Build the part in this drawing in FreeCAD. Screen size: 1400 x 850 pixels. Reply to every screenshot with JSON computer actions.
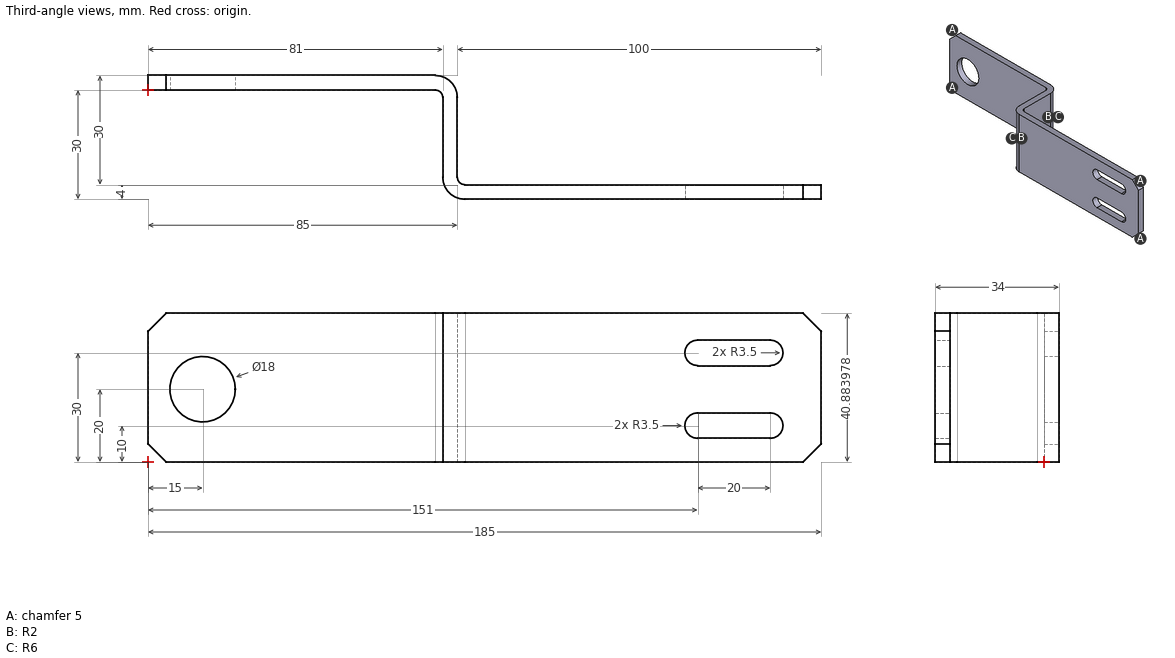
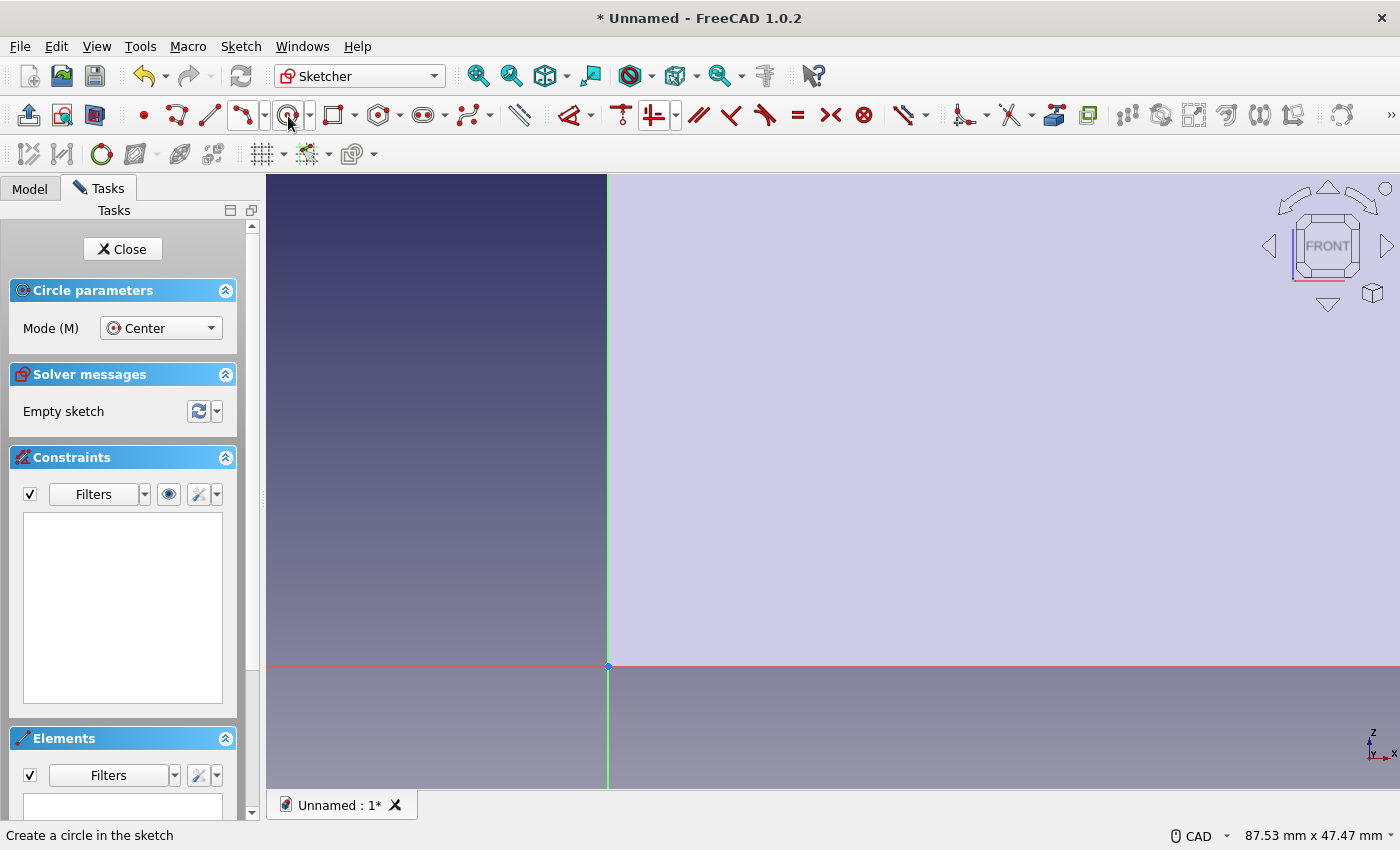
{"action": "left_click", "coordinate": [803, 408]}
{"action": "left_click", "coordinate": [885, 325]}
{"action": "key", "text": "Escape"}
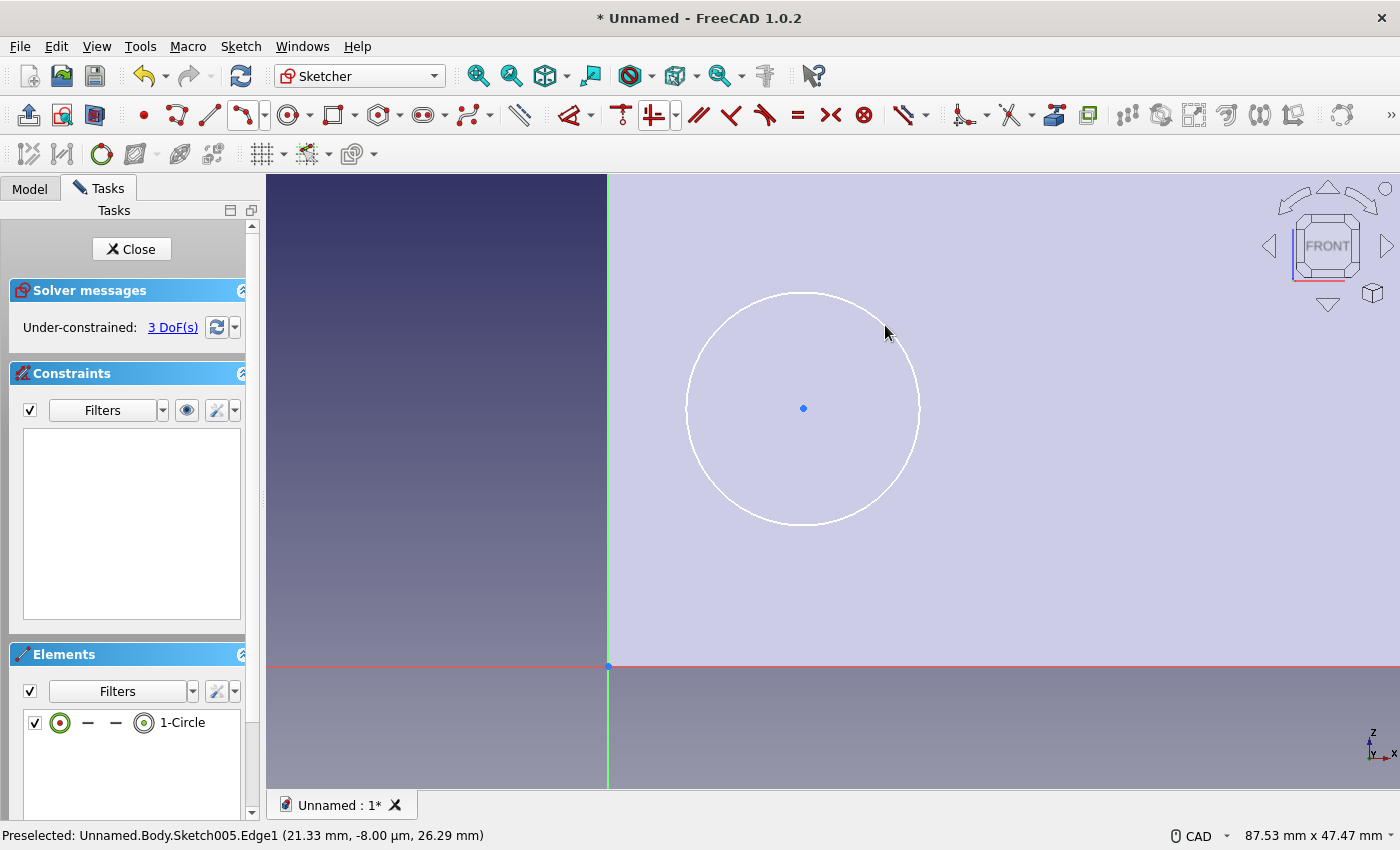
{"action": "key", "text": "d"}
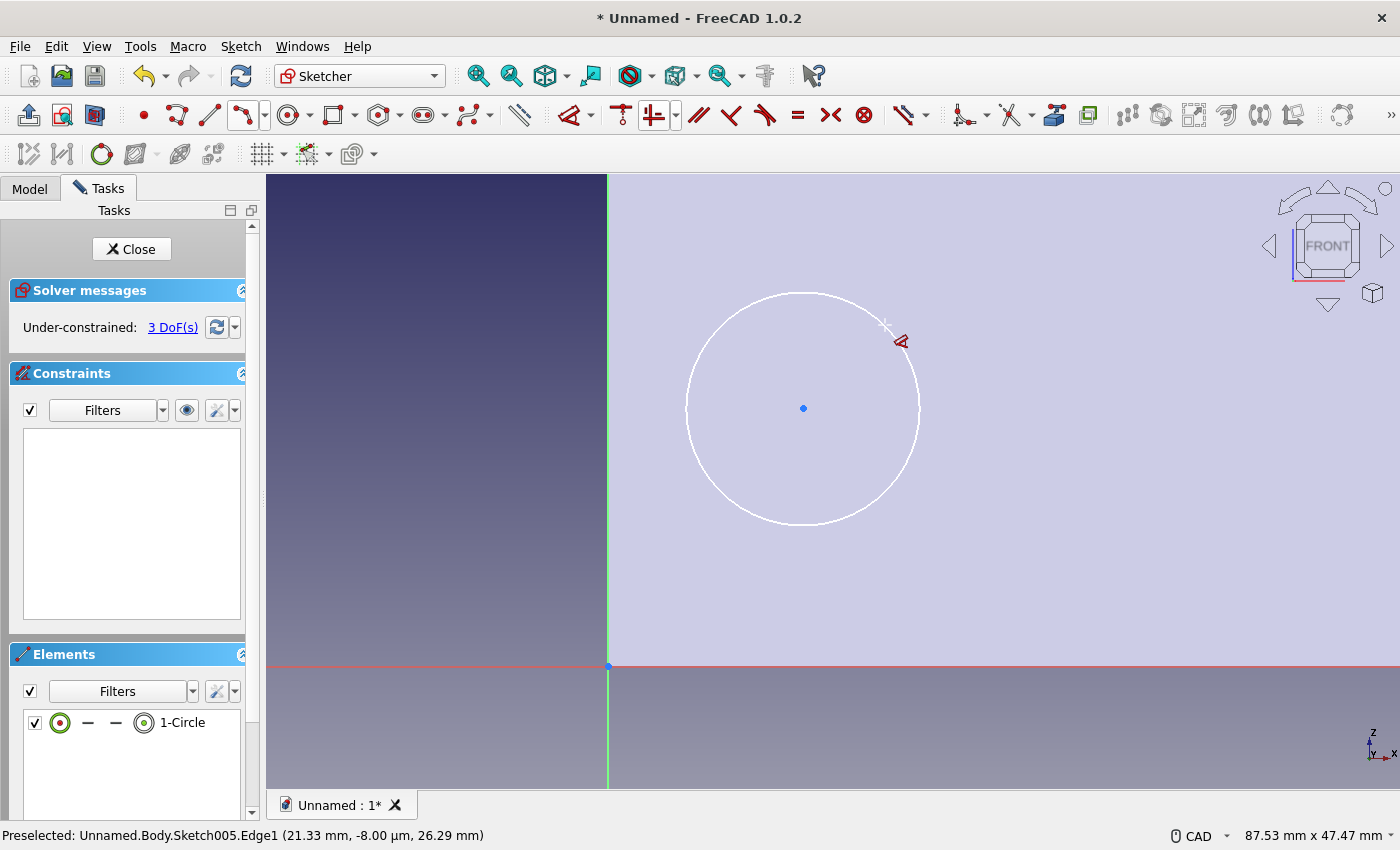
{"action": "left_click", "coordinate": [885, 326]}
{"action": "left_click", "coordinate": [907, 303]}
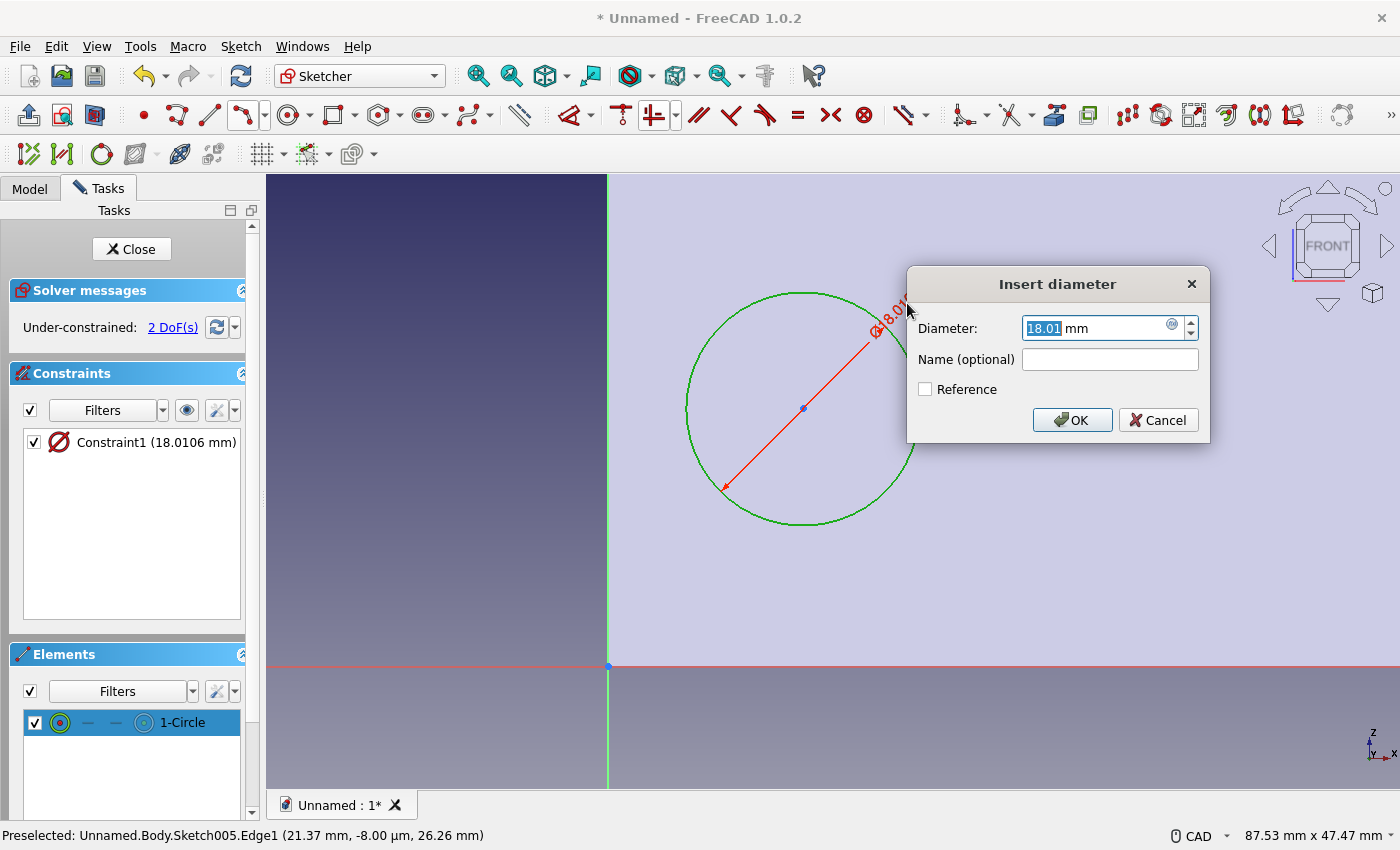
{"action": "type", "text": "18"}
{"action": "key", "text": "Return"}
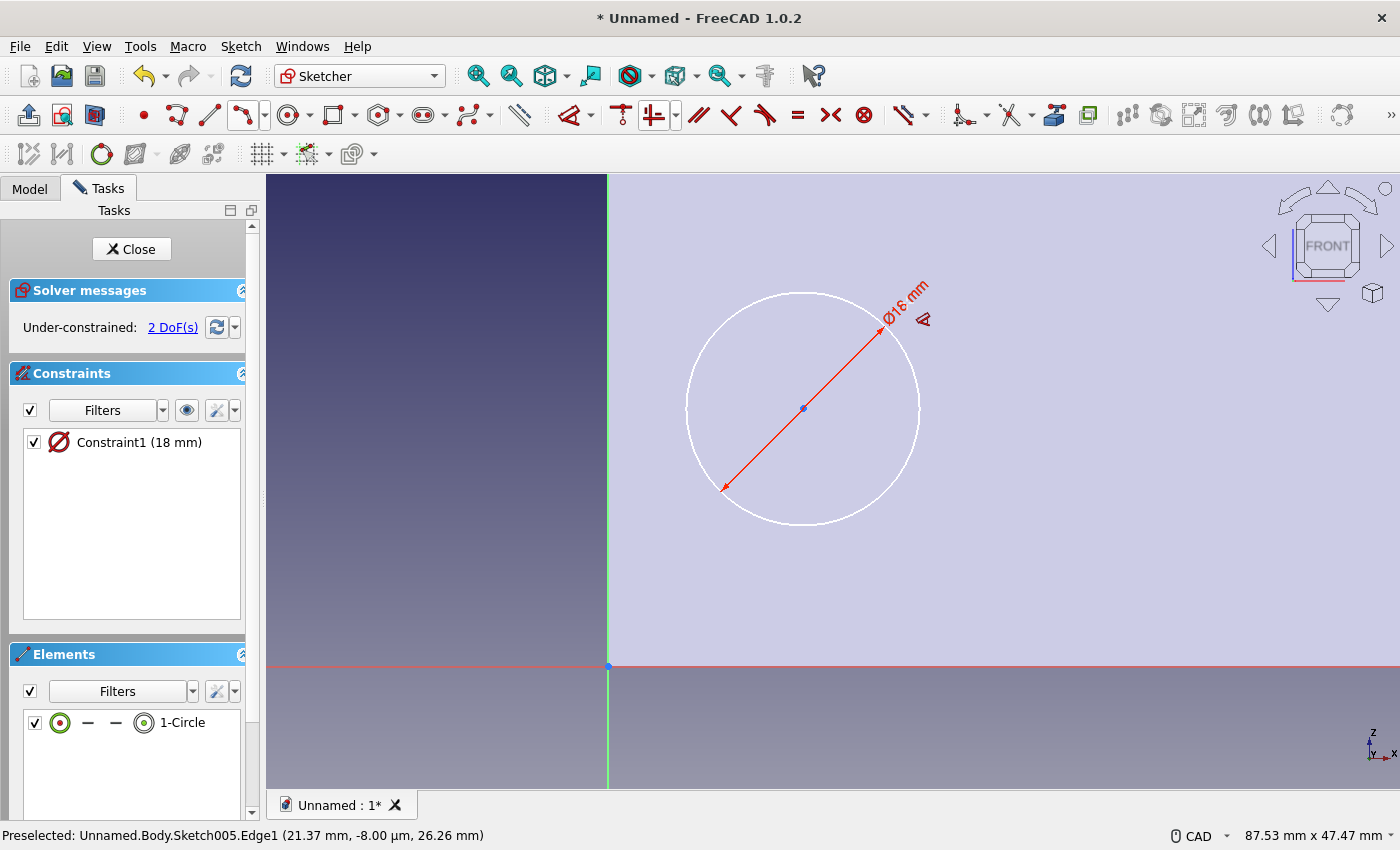
{"action": "left_click", "coordinate": [803, 409]}
{"action": "left_click", "coordinate": [706, 701]}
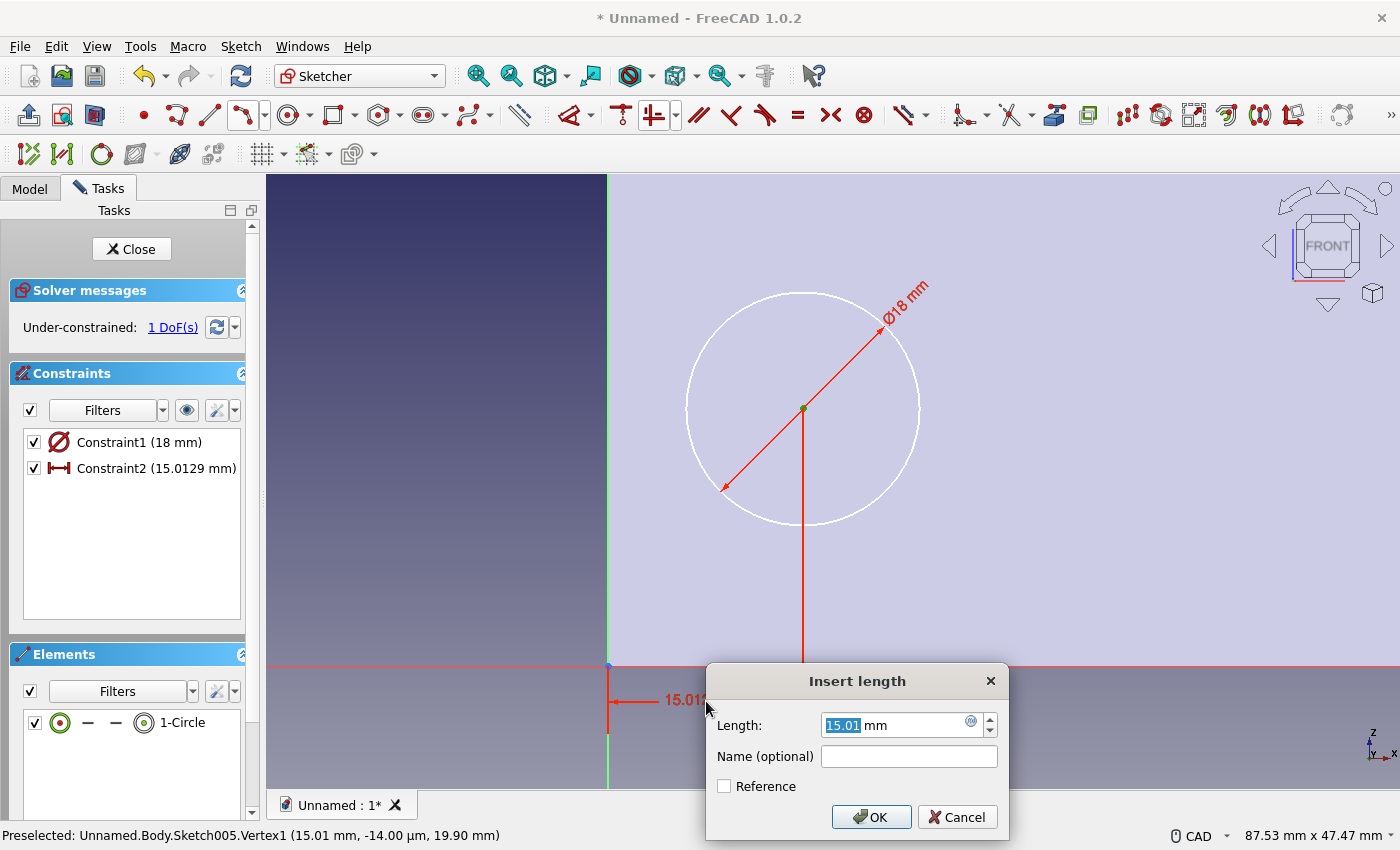
{"action": "type", "text": "15"}
{"action": "key", "text": "Return"}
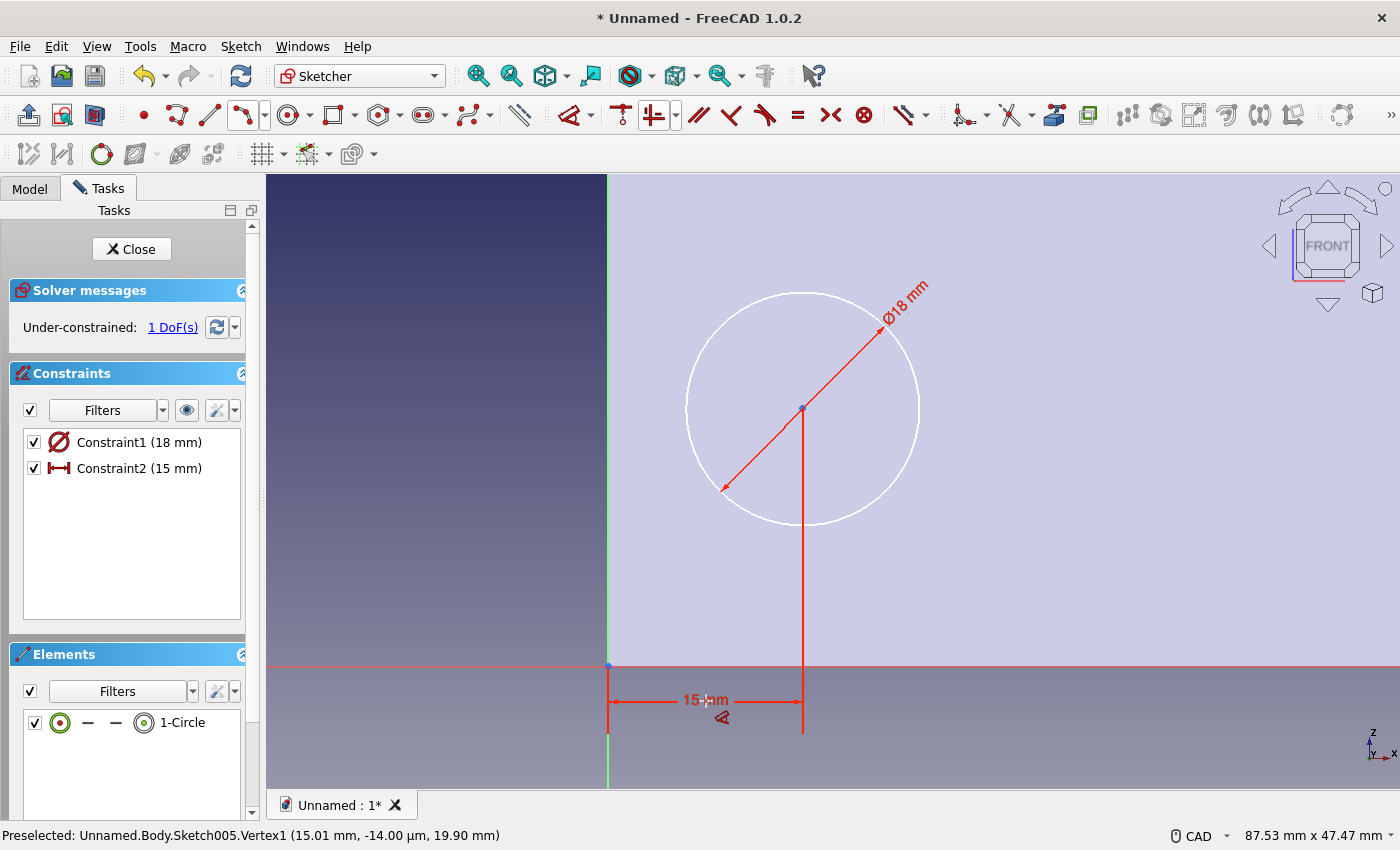
{"action": "left_click", "coordinate": [803, 409]}
{"action": "left_click", "coordinate": [574, 538]}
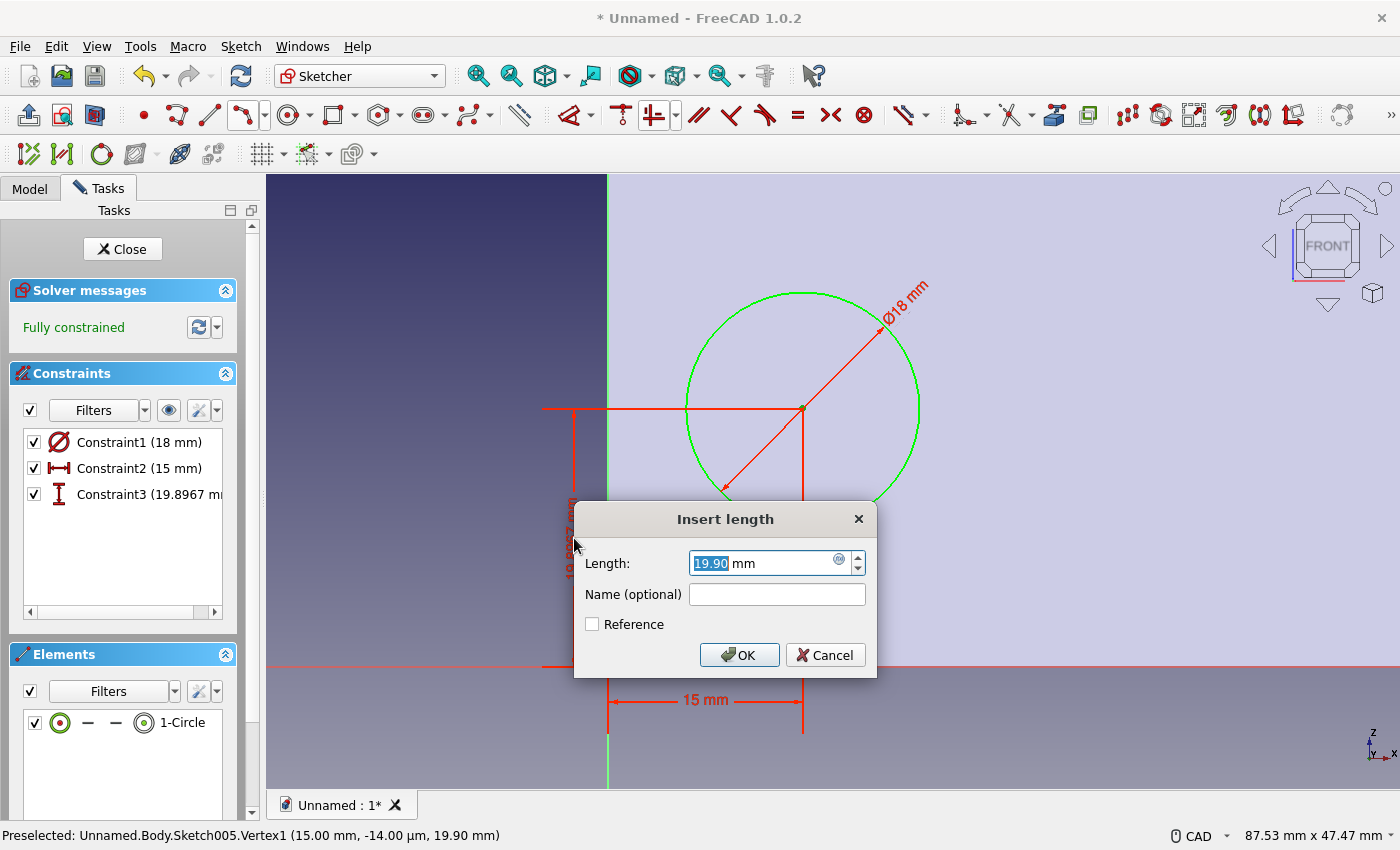
{"action": "type", "text": "20"}
{"action": "key", "text": "Return"}
{"action": "key", "text": "Escape"}